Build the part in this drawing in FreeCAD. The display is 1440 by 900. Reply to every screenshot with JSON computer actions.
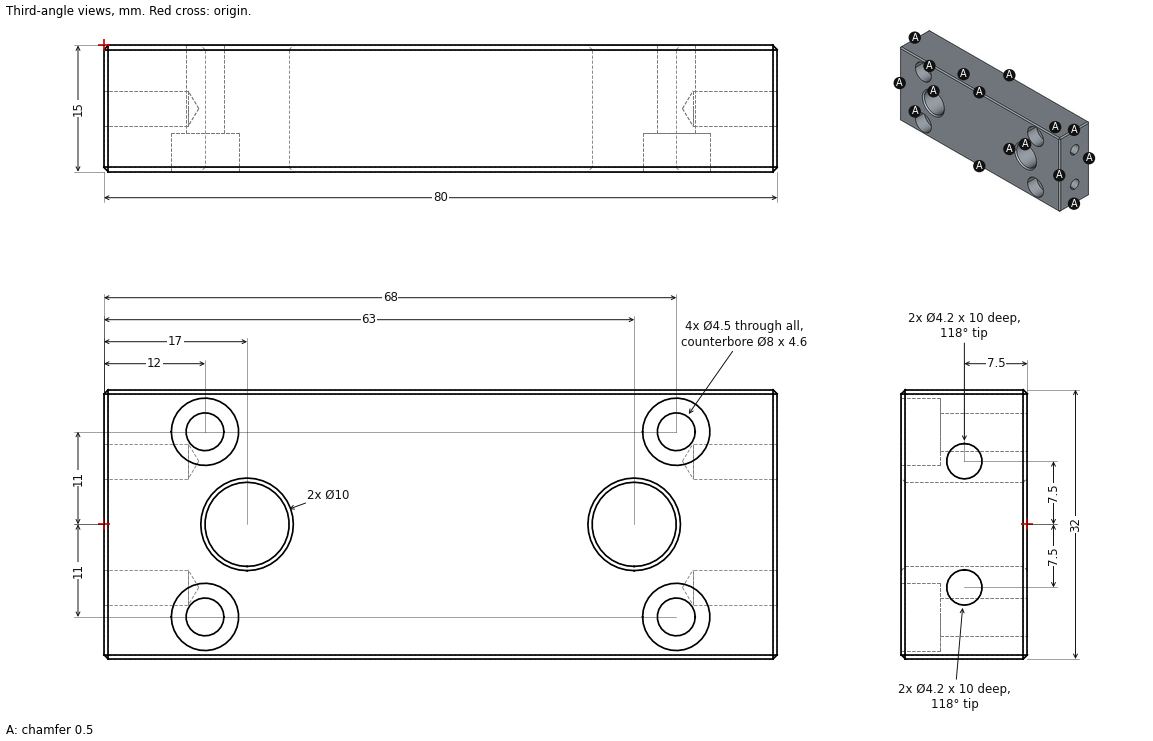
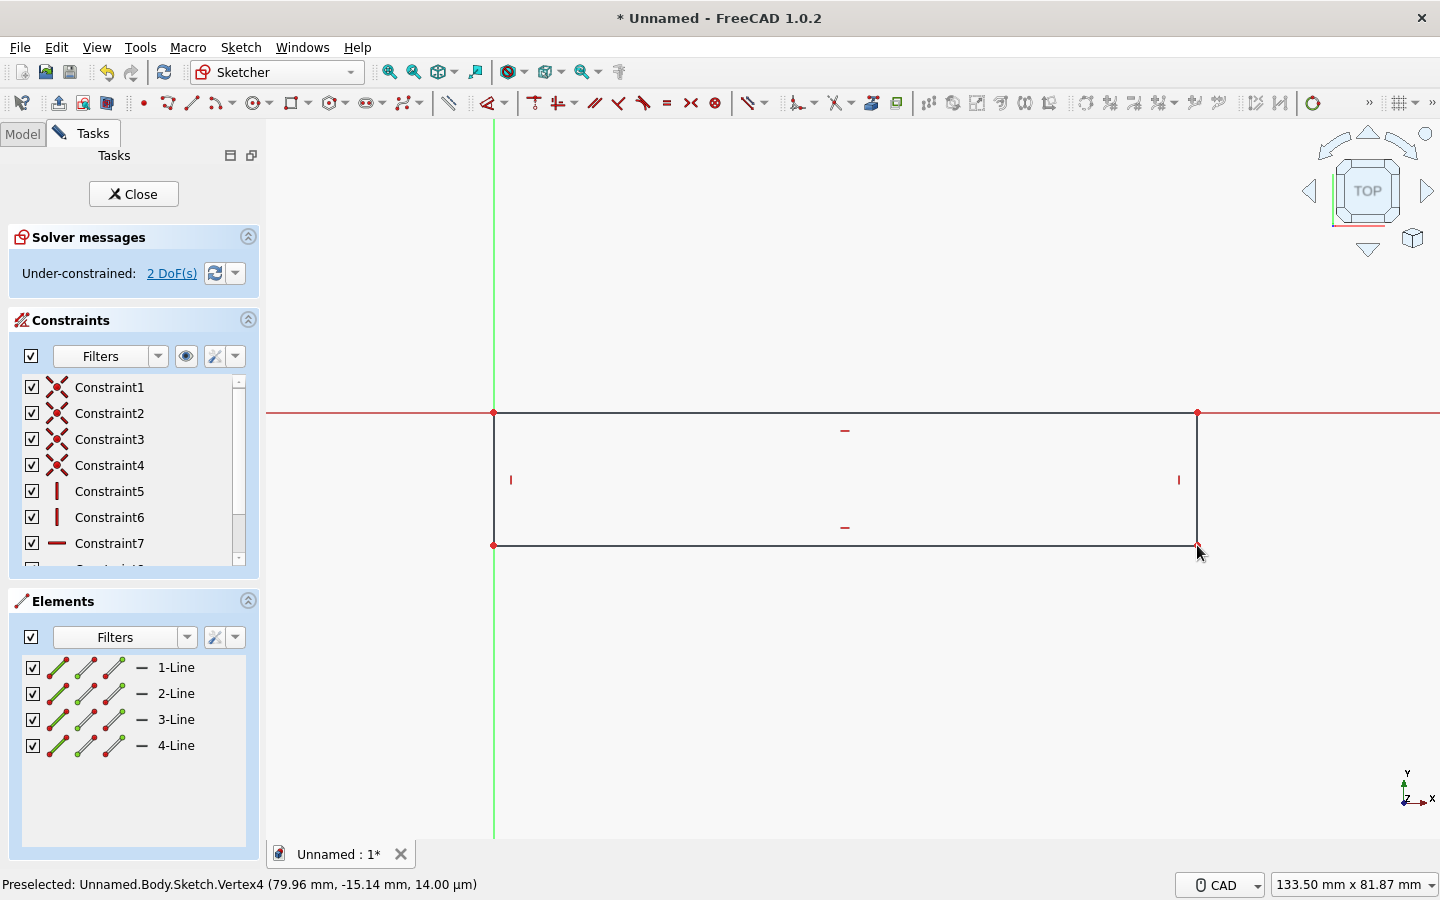
{"action": "left_click", "coordinate": [494, 453]}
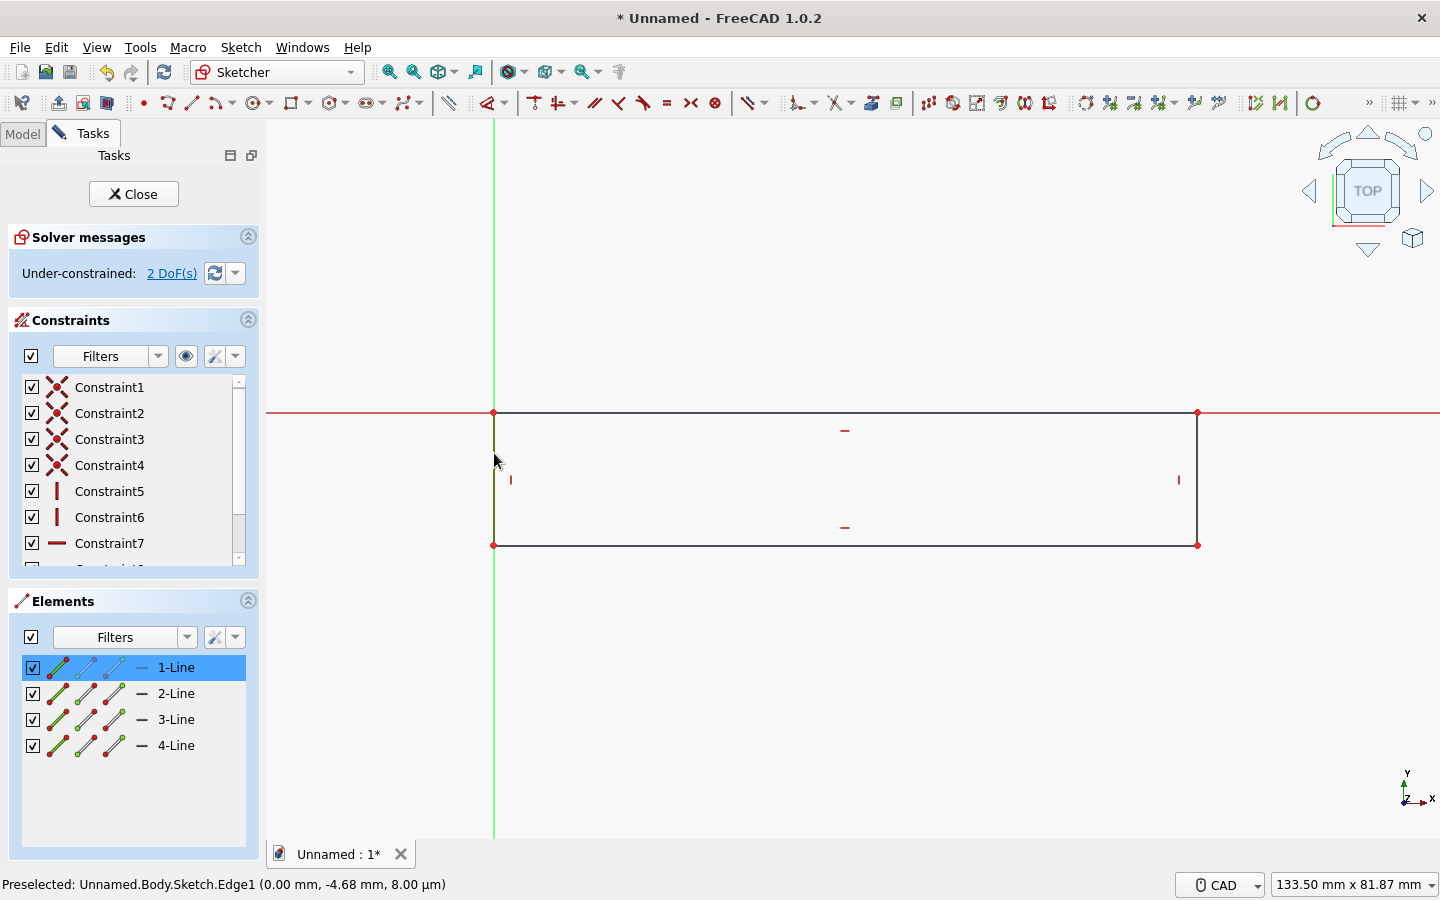
{"action": "left_click", "coordinate": [506, 104]}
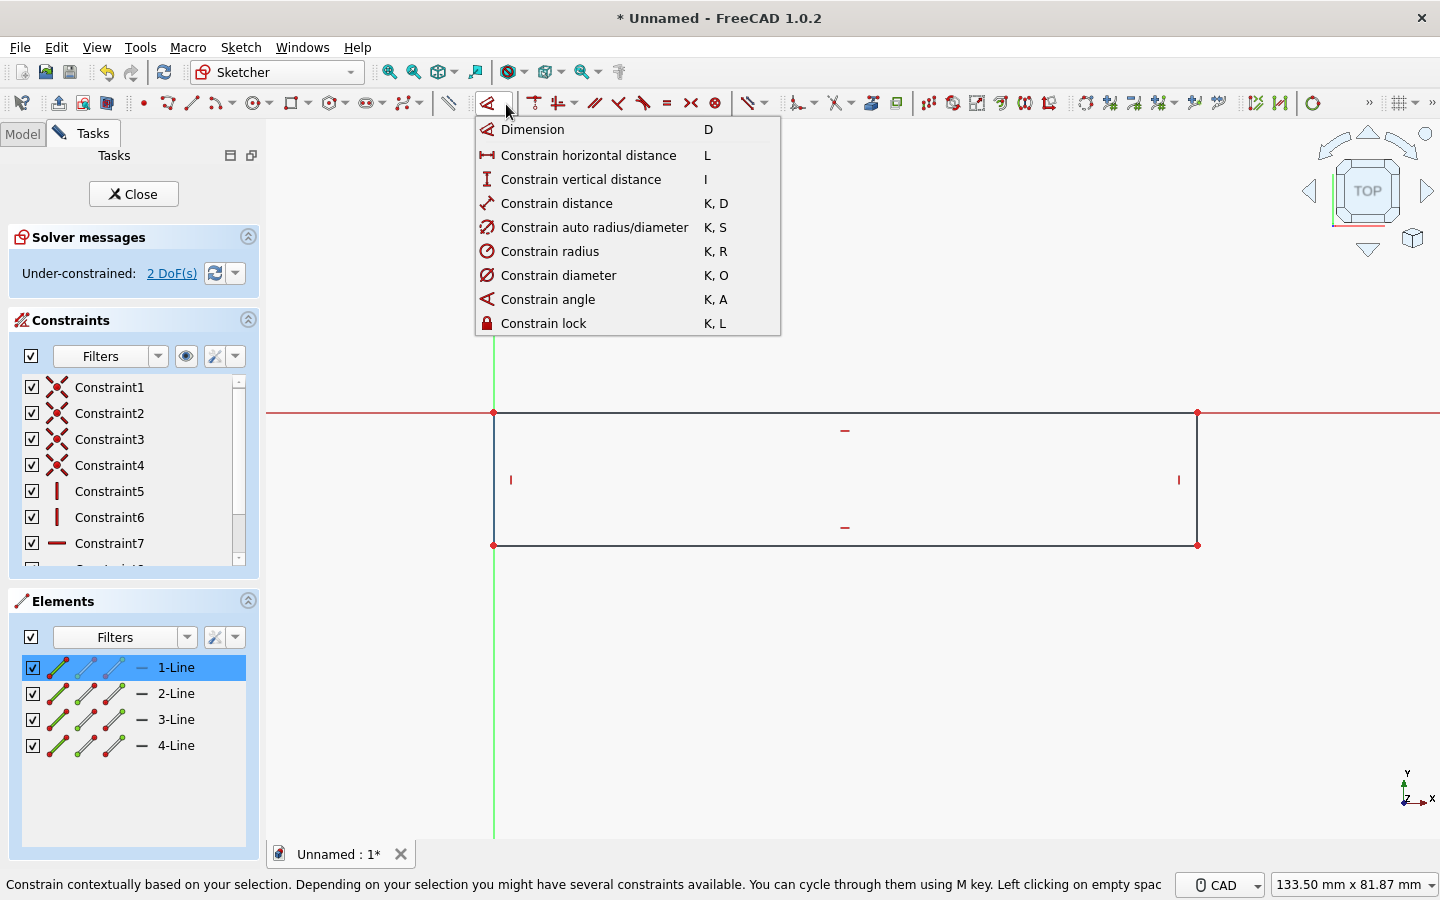
{"action": "left_click", "coordinate": [628, 179]}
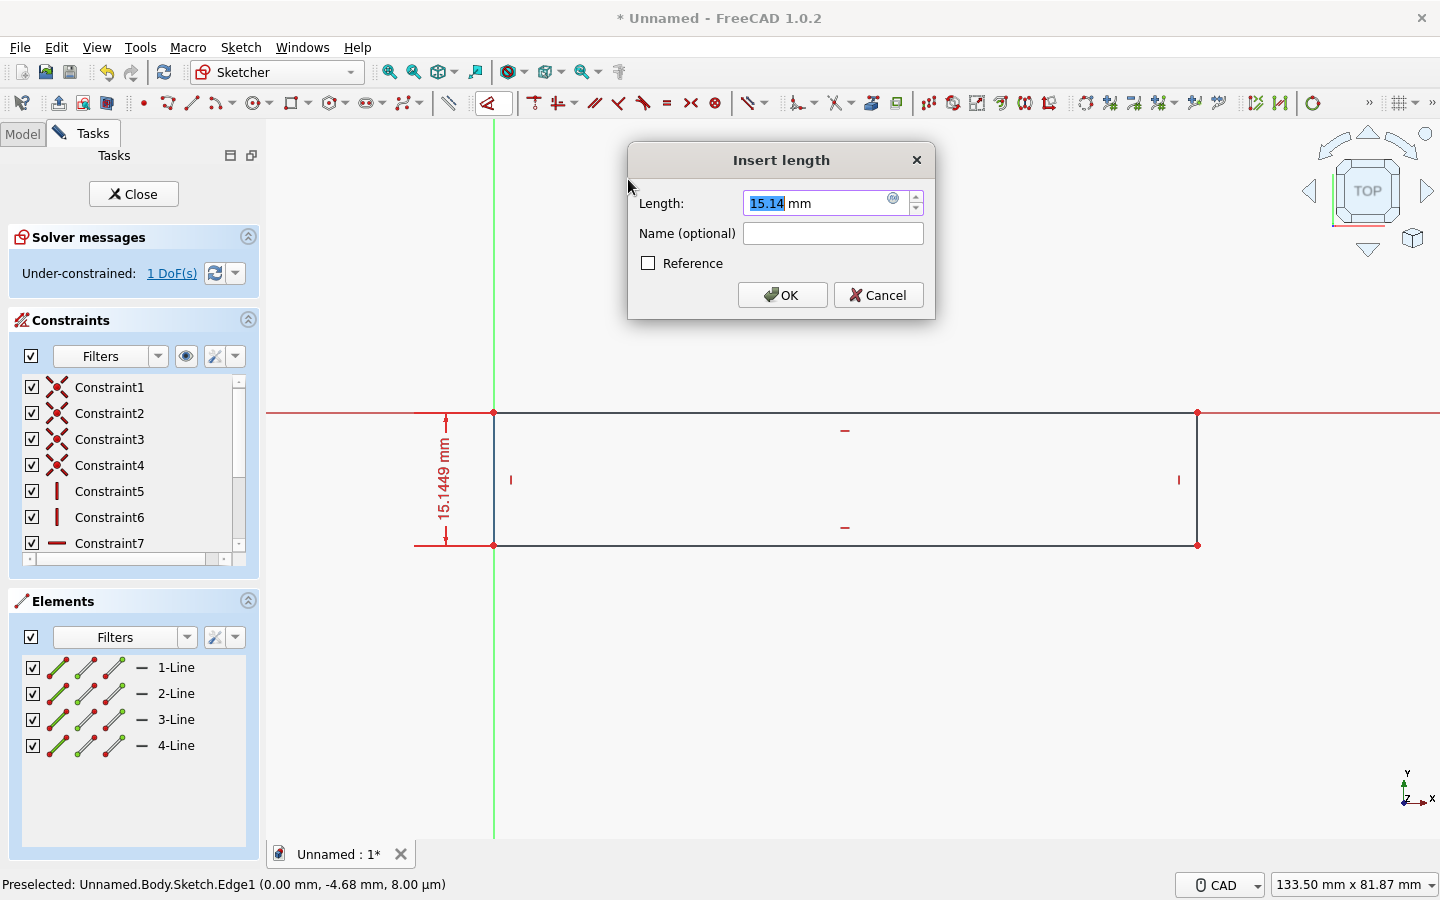
{"action": "type", "text": "15"}
{"action": "key", "text": "Return"}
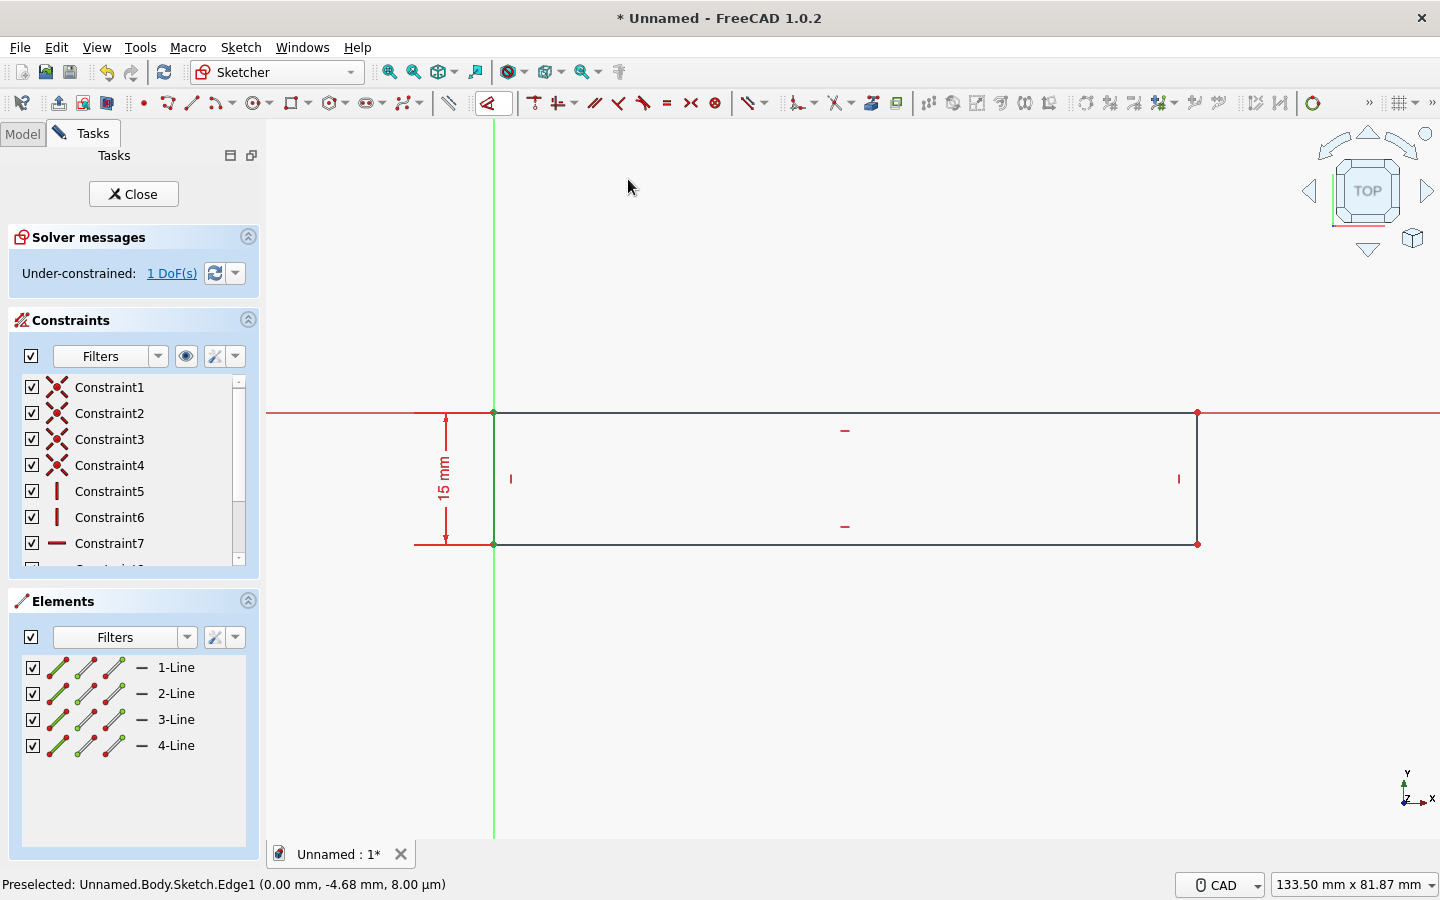
{"action": "left_click", "coordinate": [705, 545]}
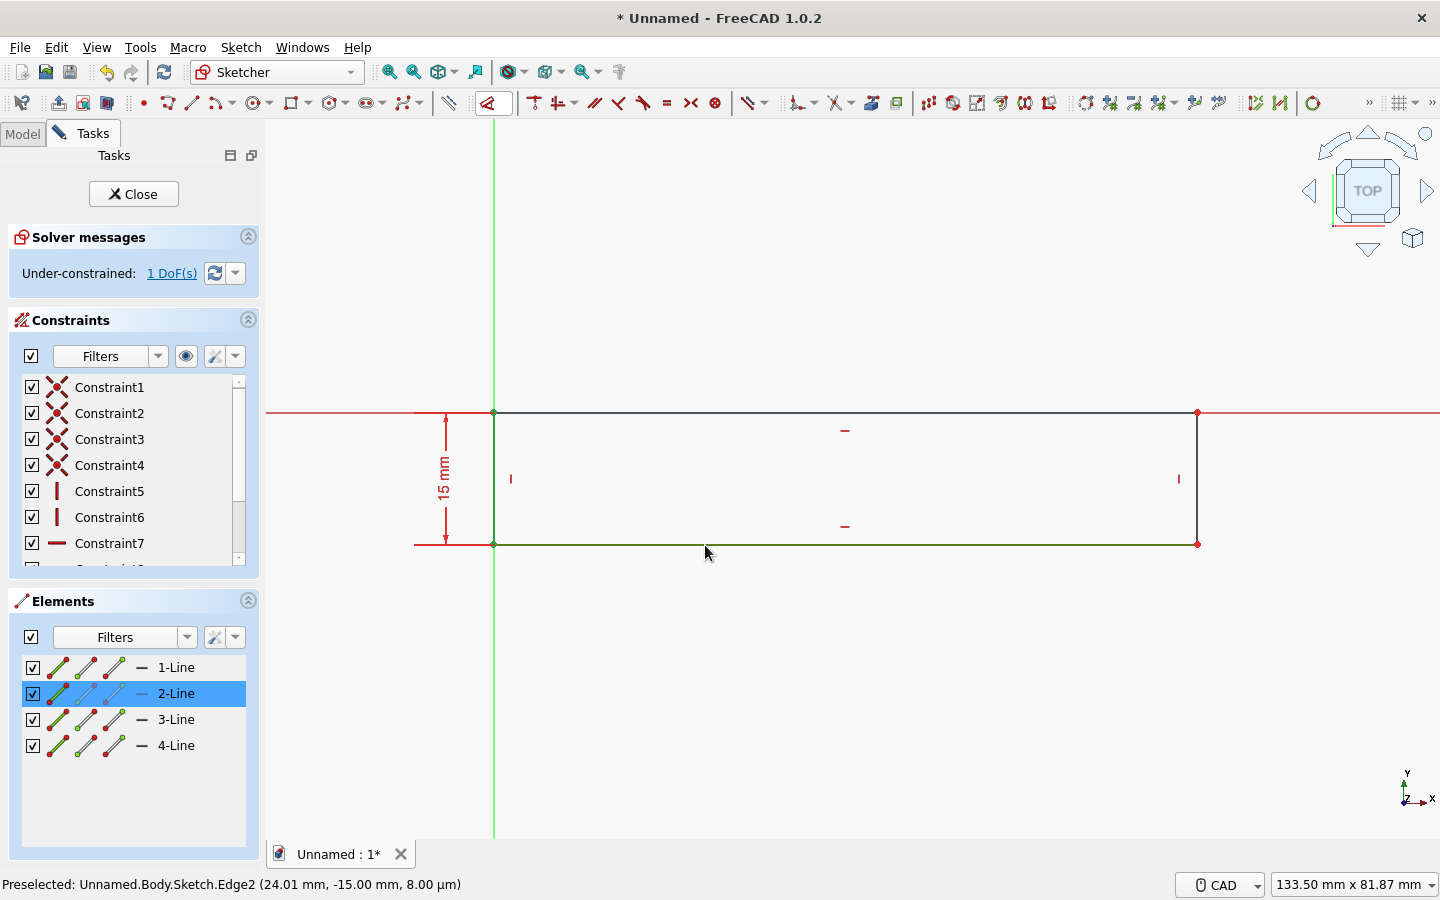
{"action": "left_click", "coordinate": [506, 104]}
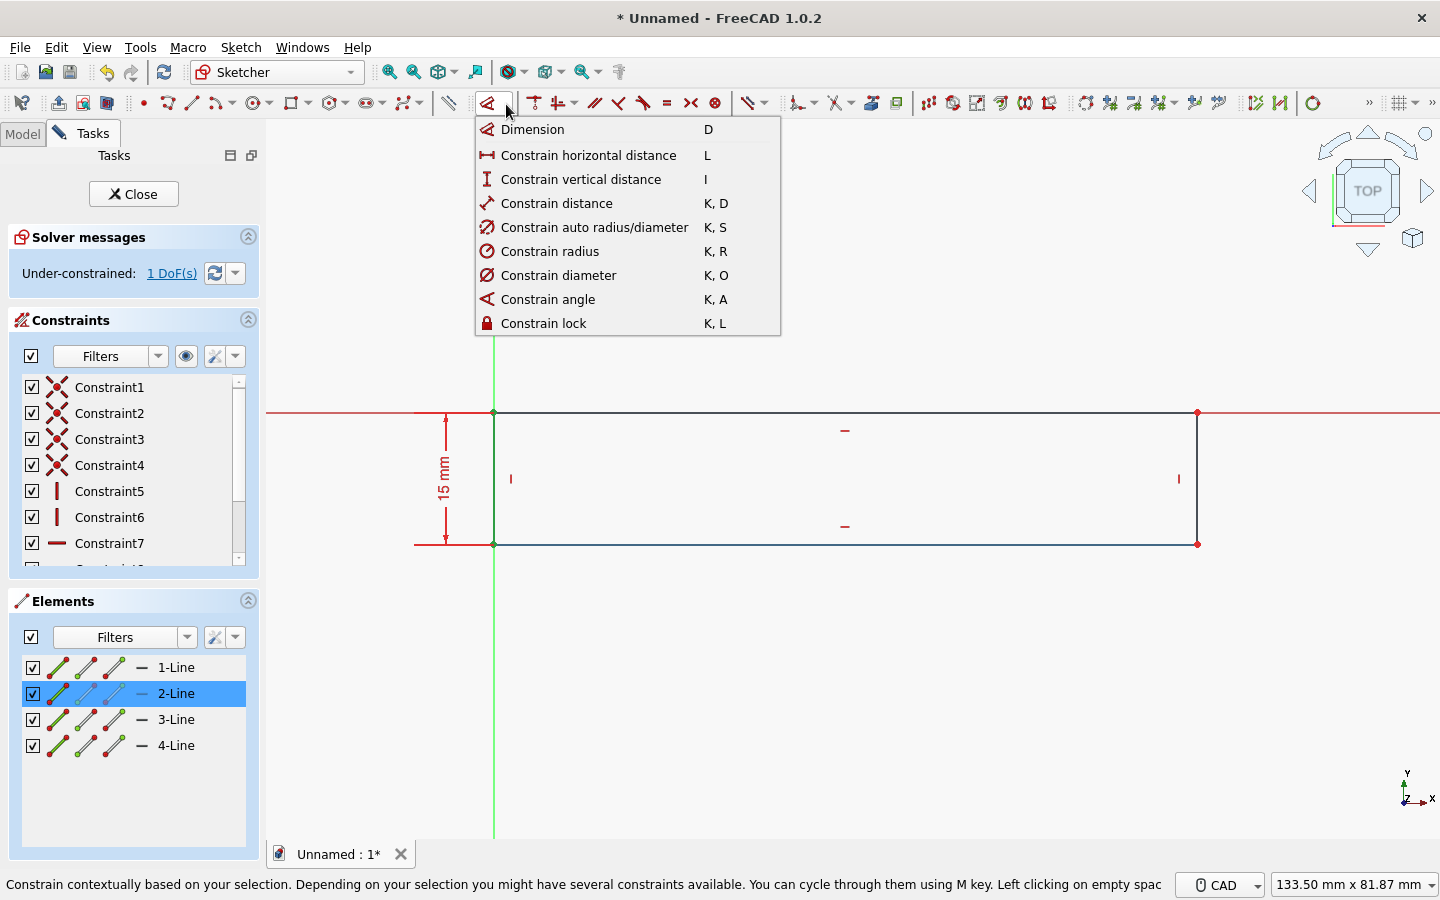
{"action": "left_click", "coordinate": [628, 155]}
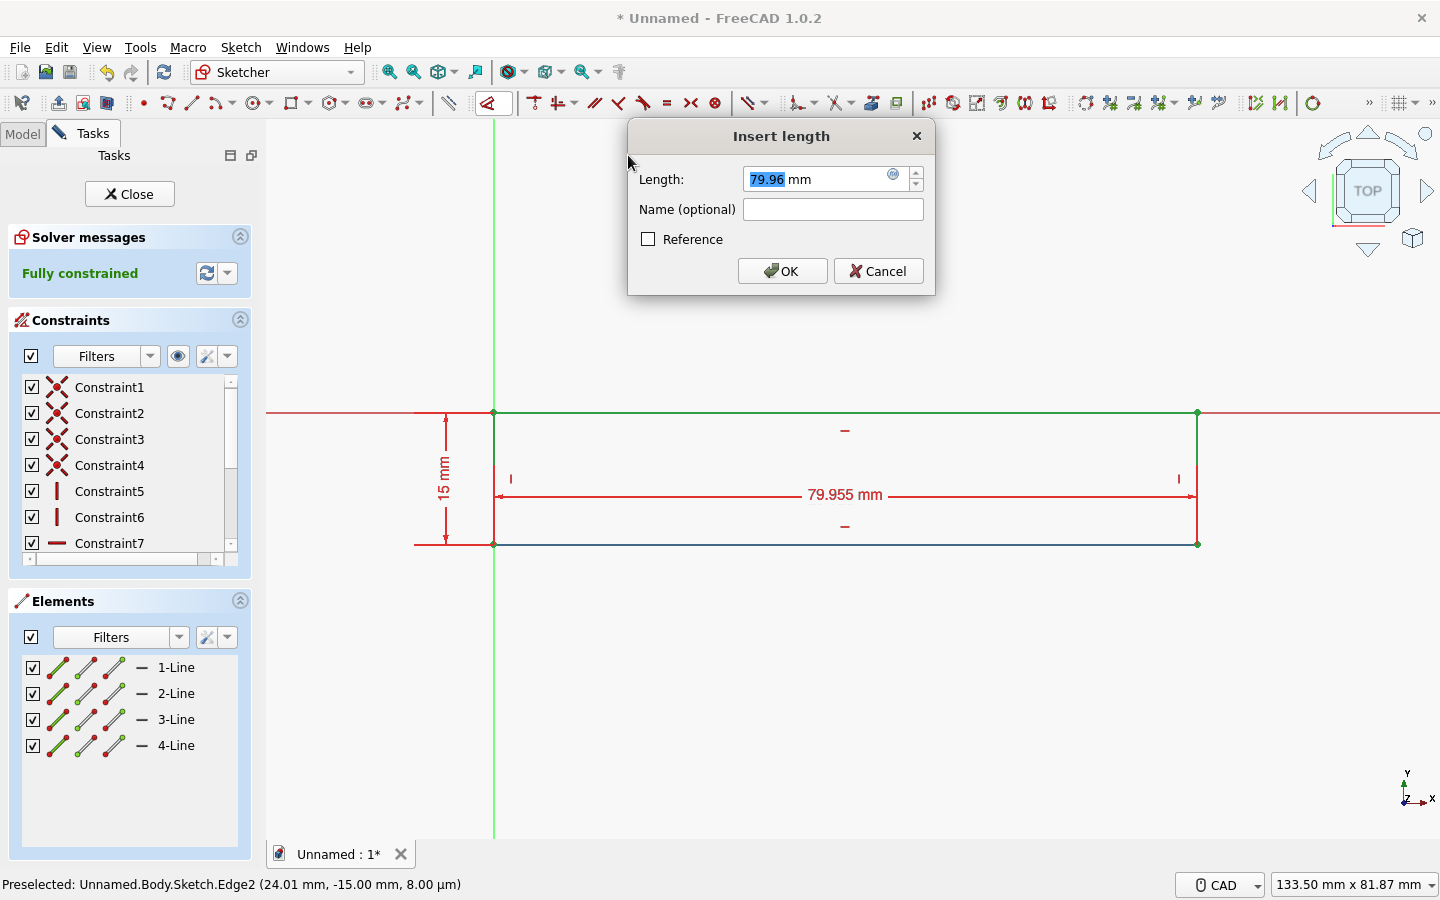
{"action": "type", "text": "80"}
{"action": "key", "text": "Return"}